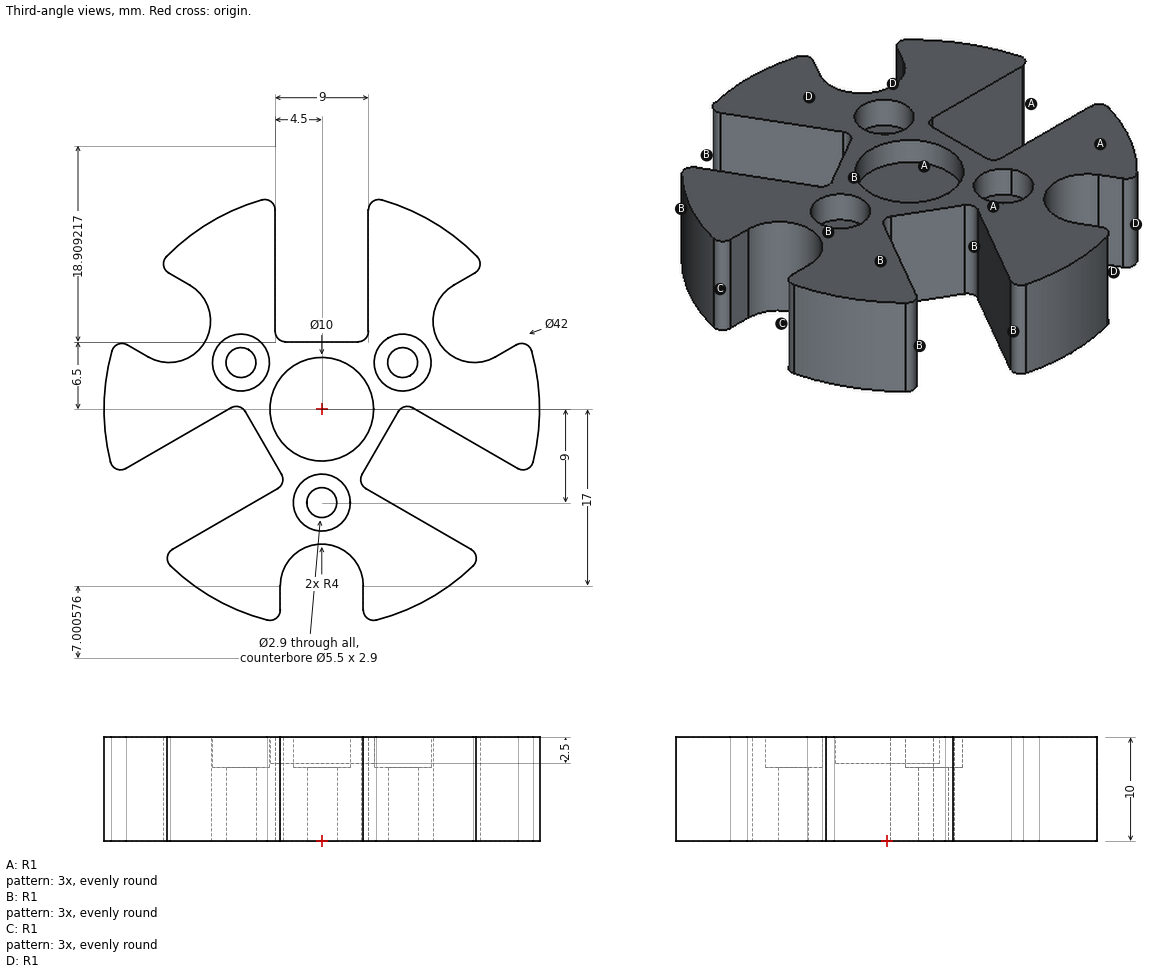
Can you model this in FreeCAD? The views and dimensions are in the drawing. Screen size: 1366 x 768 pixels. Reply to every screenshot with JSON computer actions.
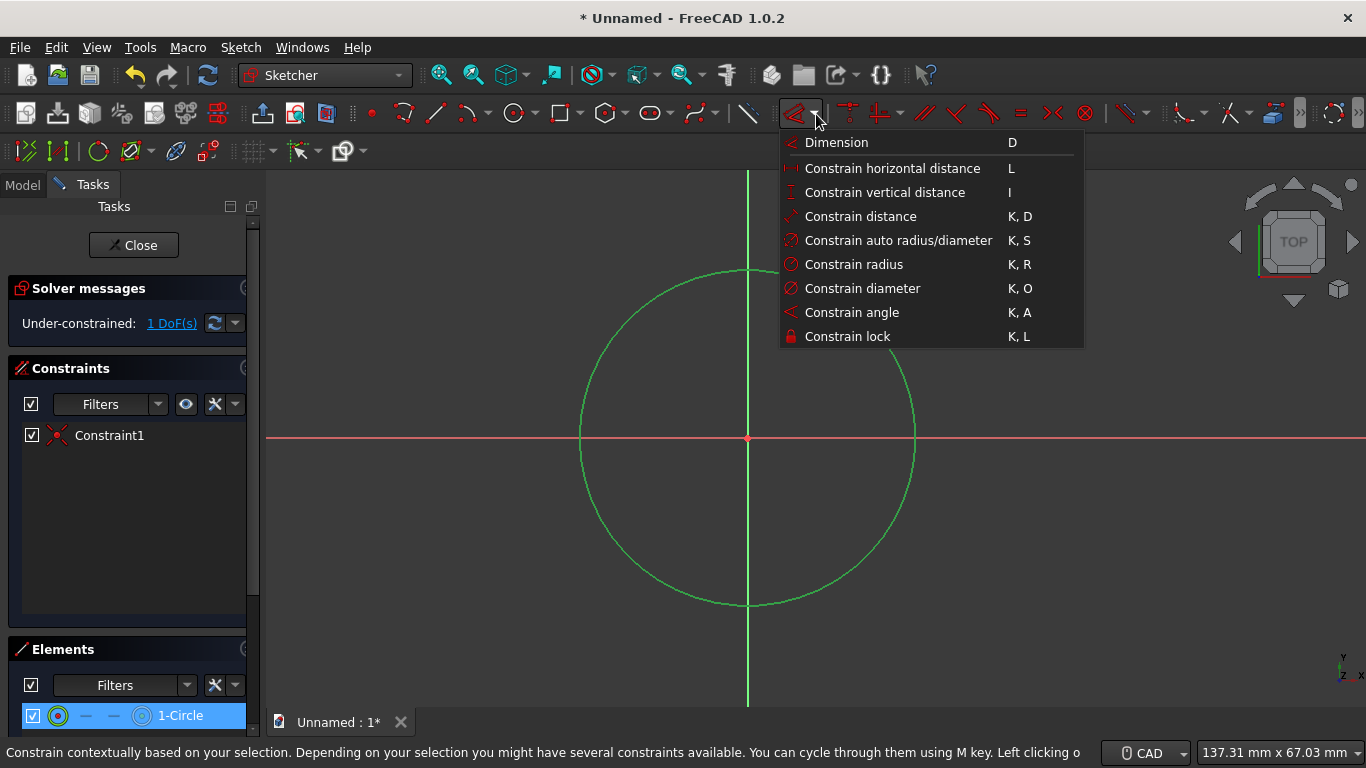
{"action": "left_click", "coordinate": [932, 288]}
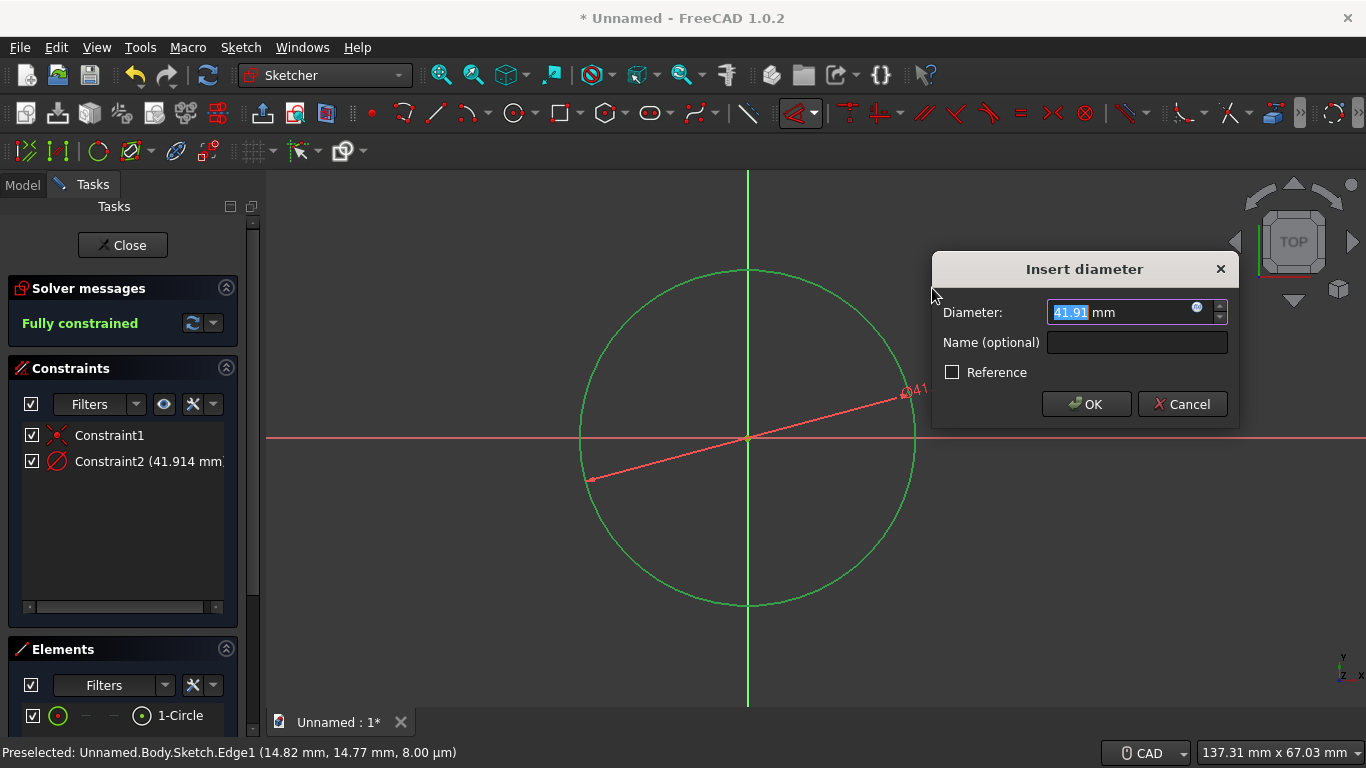
{"action": "type", "text": "42"}
{"action": "key", "text": "Return"}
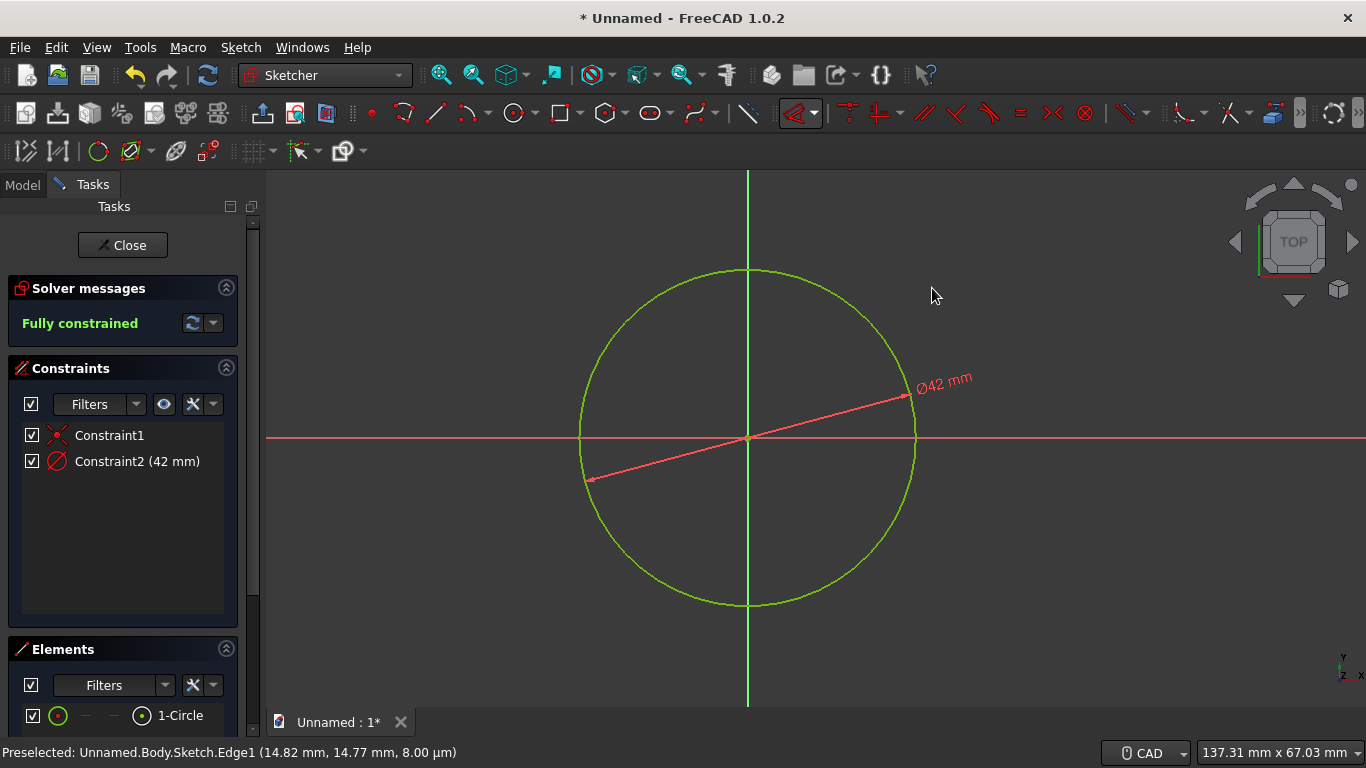
{"action": "left_click", "coordinate": [123, 245]}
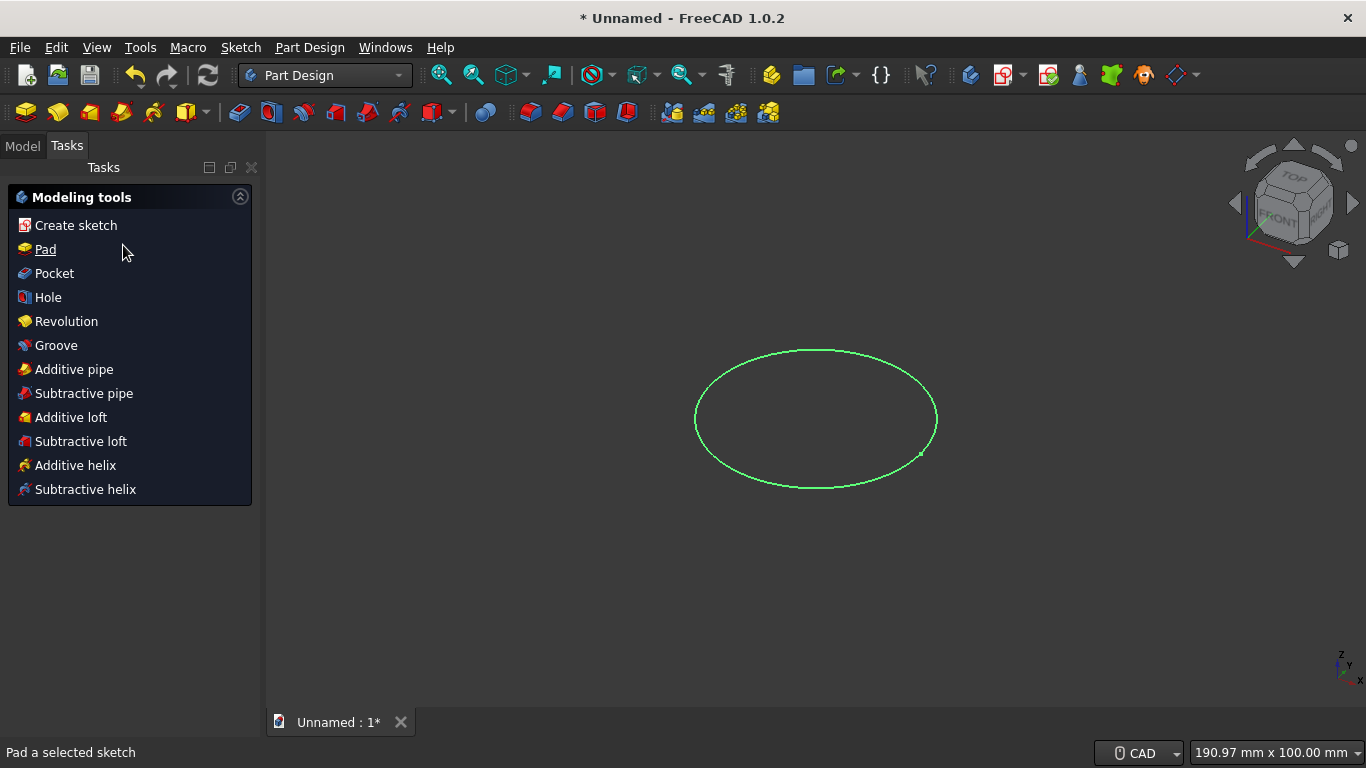
{"action": "left_click", "coordinate": [26, 112]}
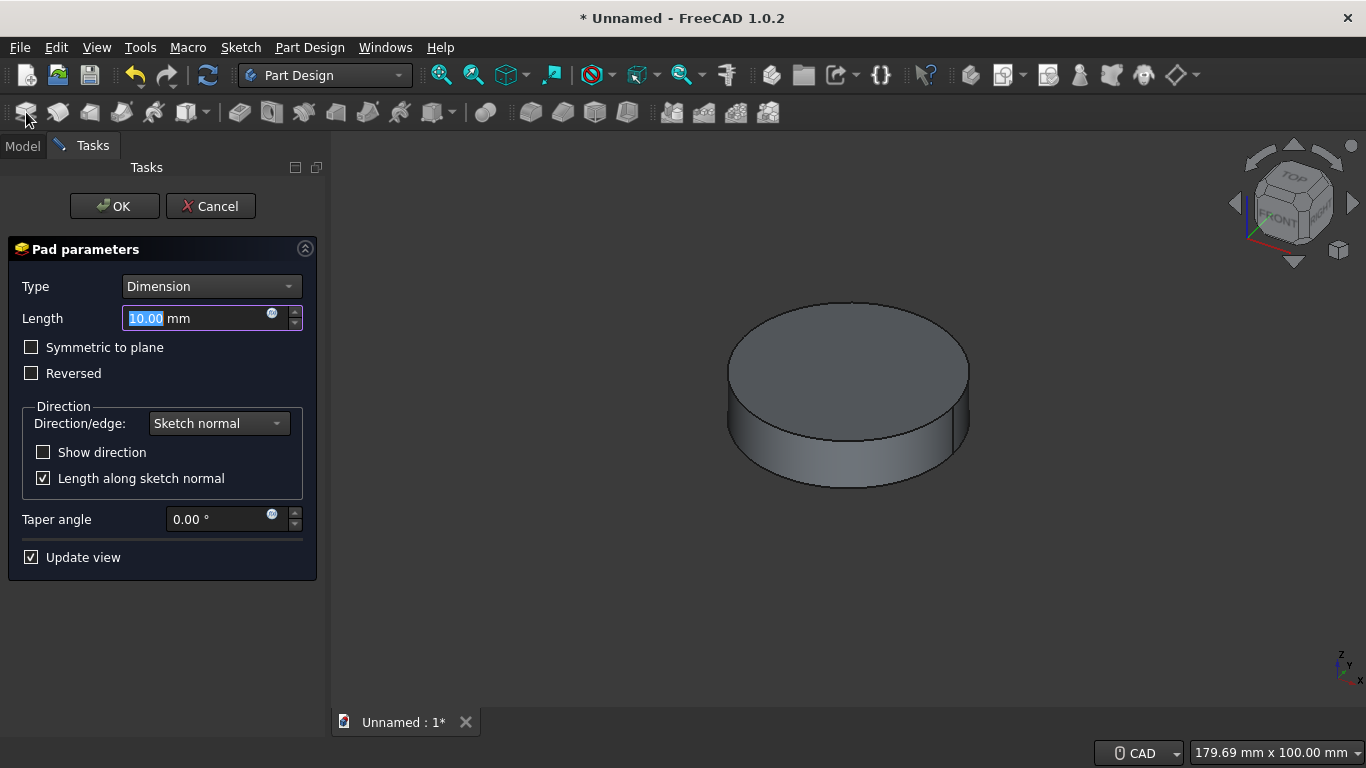
{"action": "type", "text": "10"}
{"action": "key", "text": "Tab"}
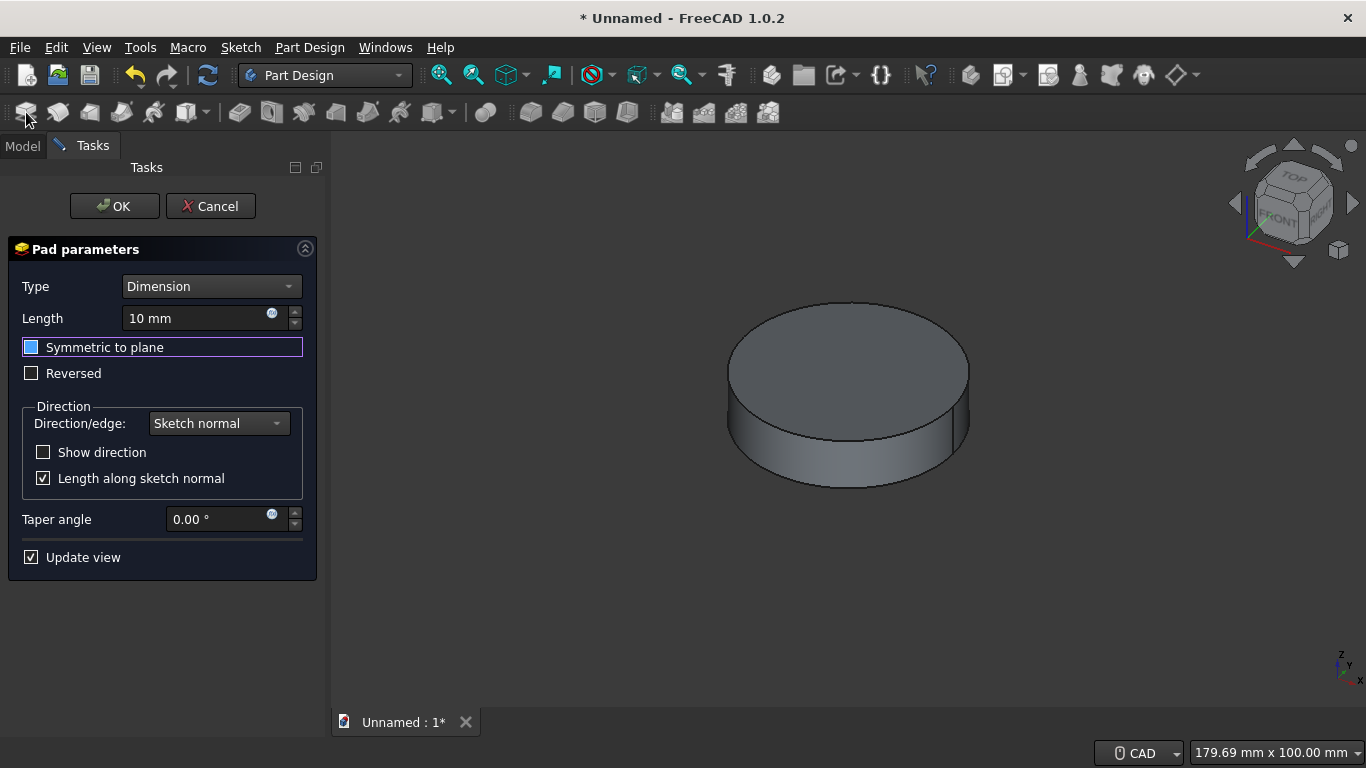
{"action": "left_click", "coordinate": [115, 206]}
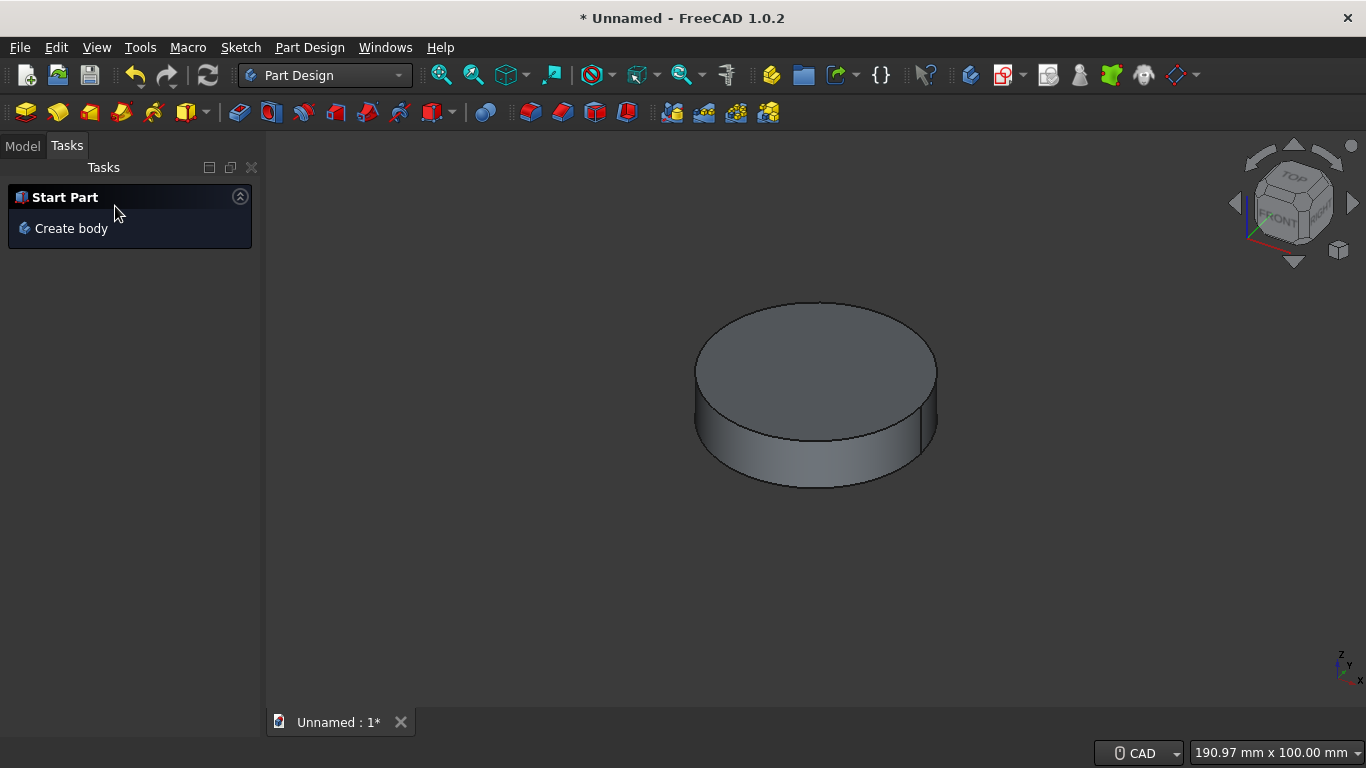
{"action": "left_click", "coordinate": [442, 76]}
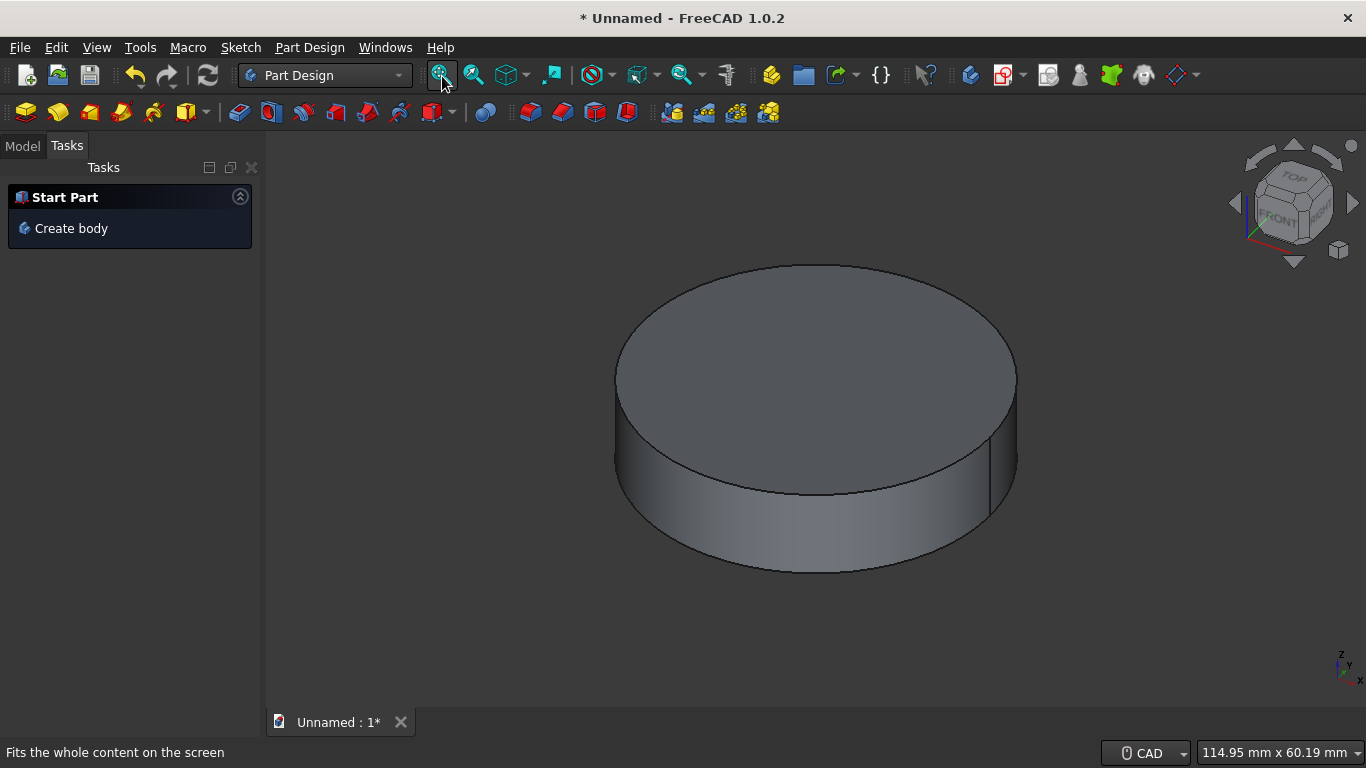
{"action": "left_click", "coordinate": [816, 379]}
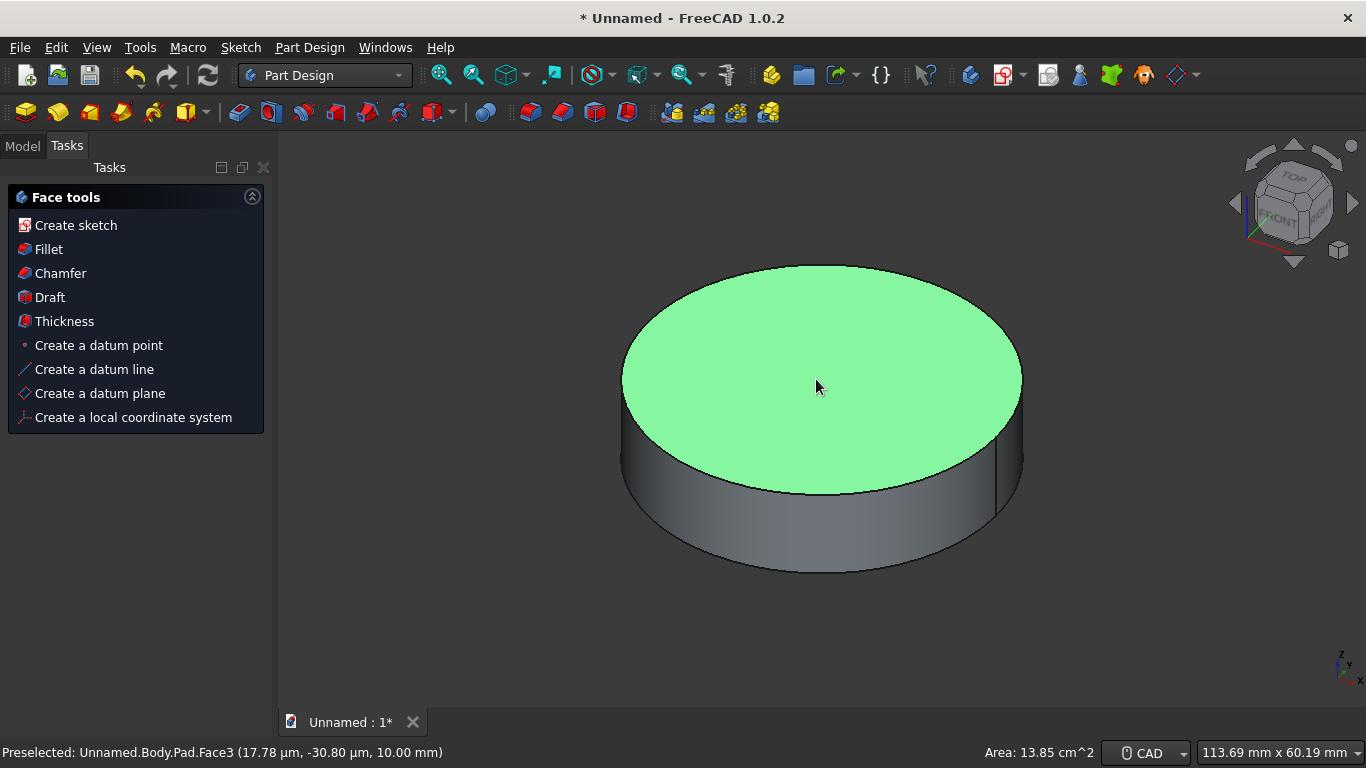
{"action": "left_click", "coordinate": [1004, 76]}